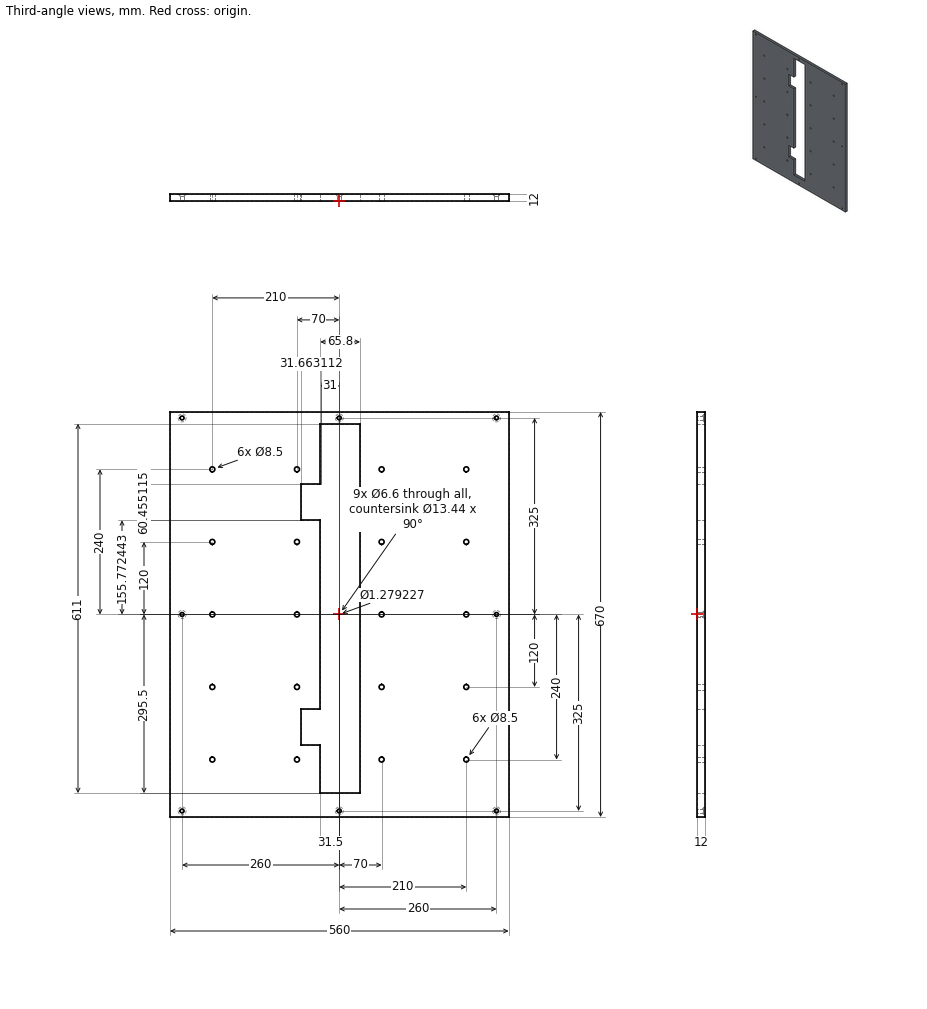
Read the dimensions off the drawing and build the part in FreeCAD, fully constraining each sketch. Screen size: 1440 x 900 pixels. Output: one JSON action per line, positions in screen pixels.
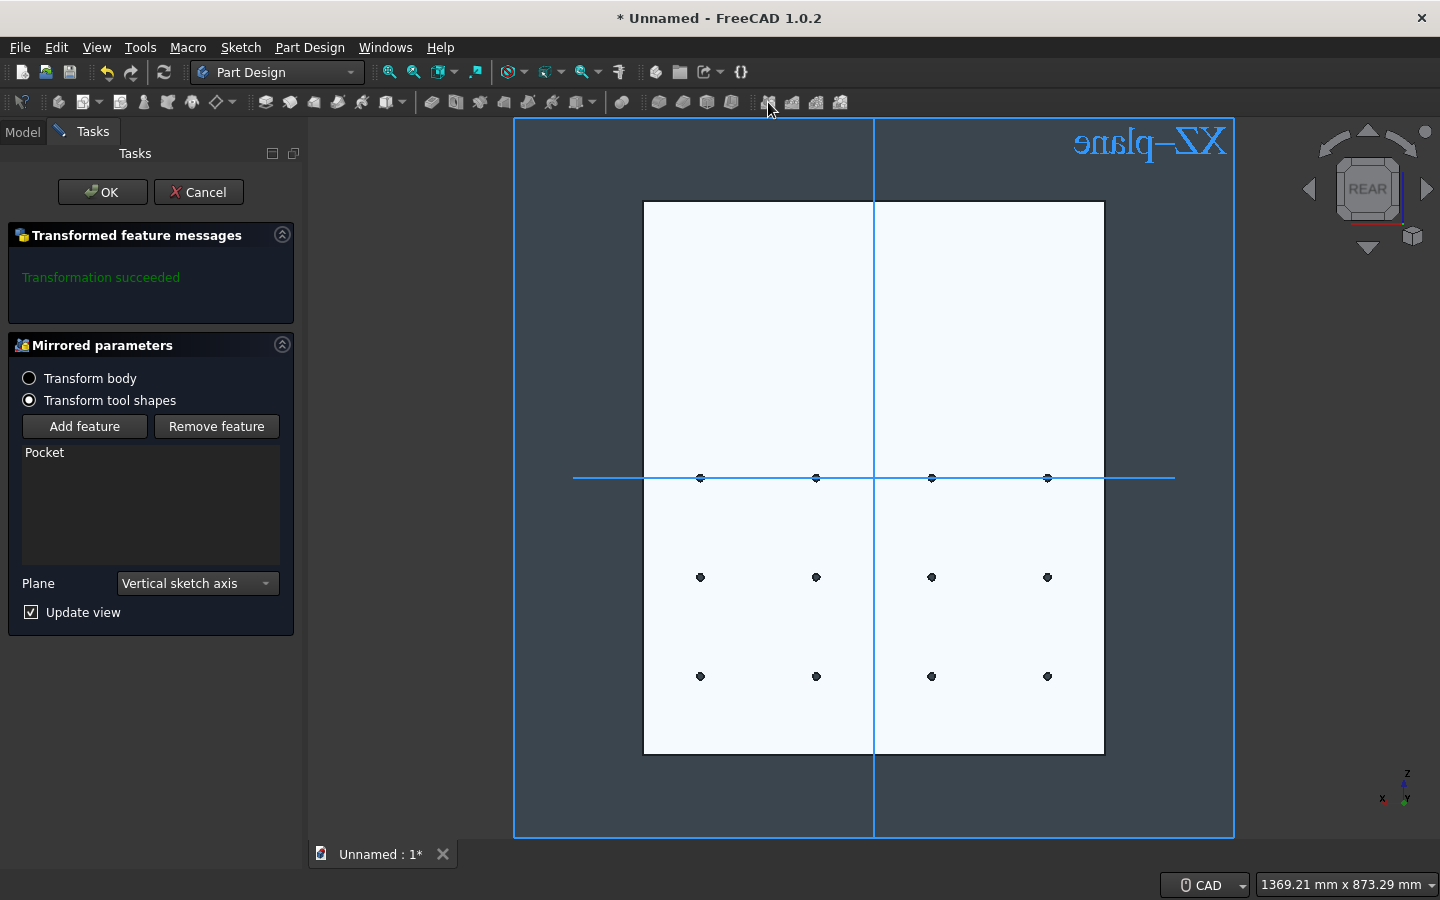
{"action": "left_click", "coordinate": [198, 584]}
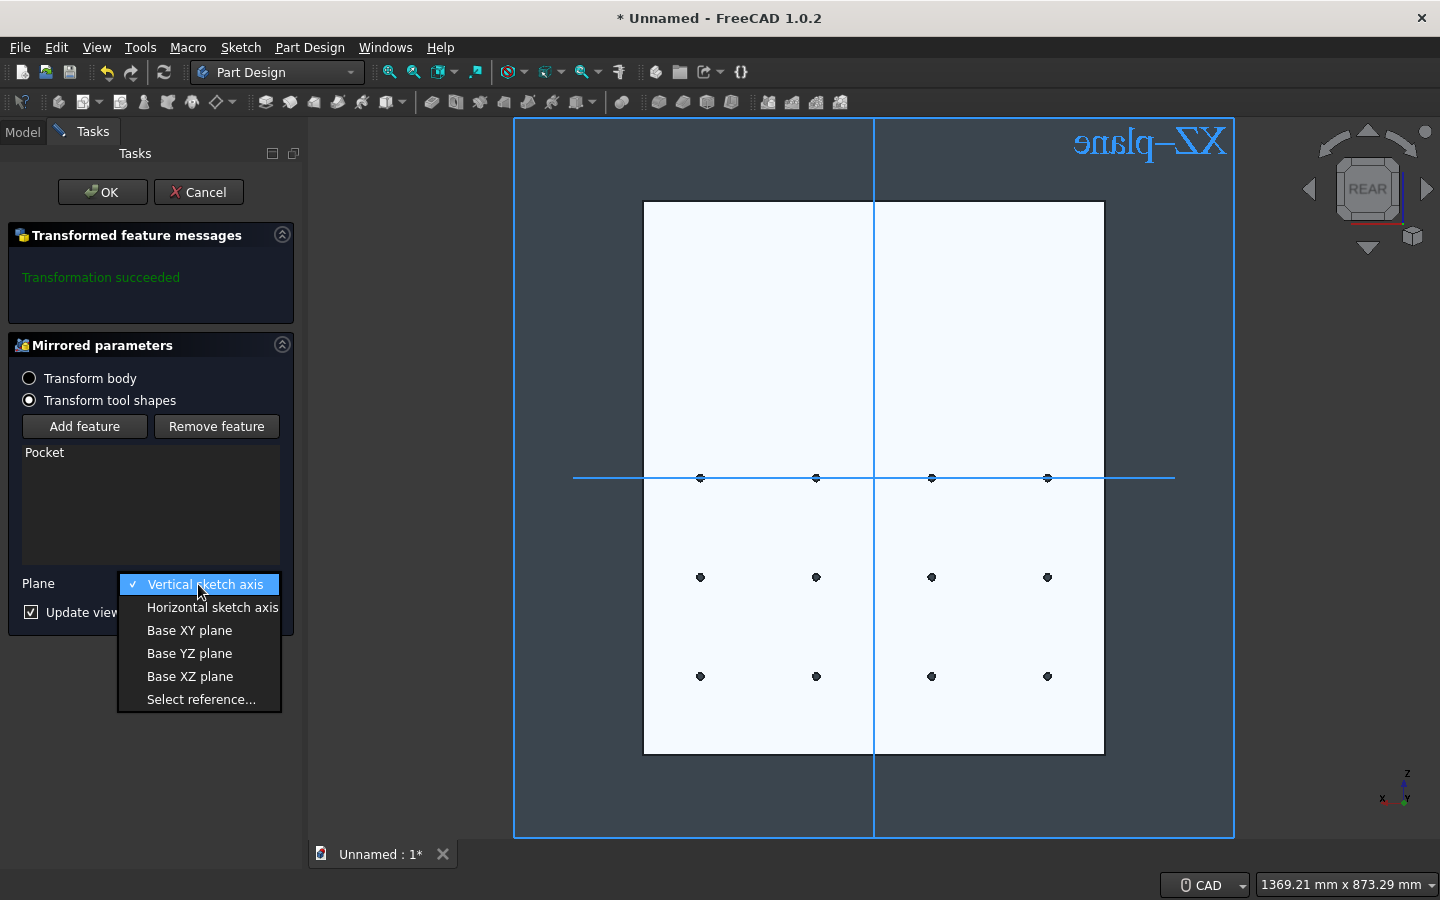
{"action": "left_click", "coordinate": [198, 630]}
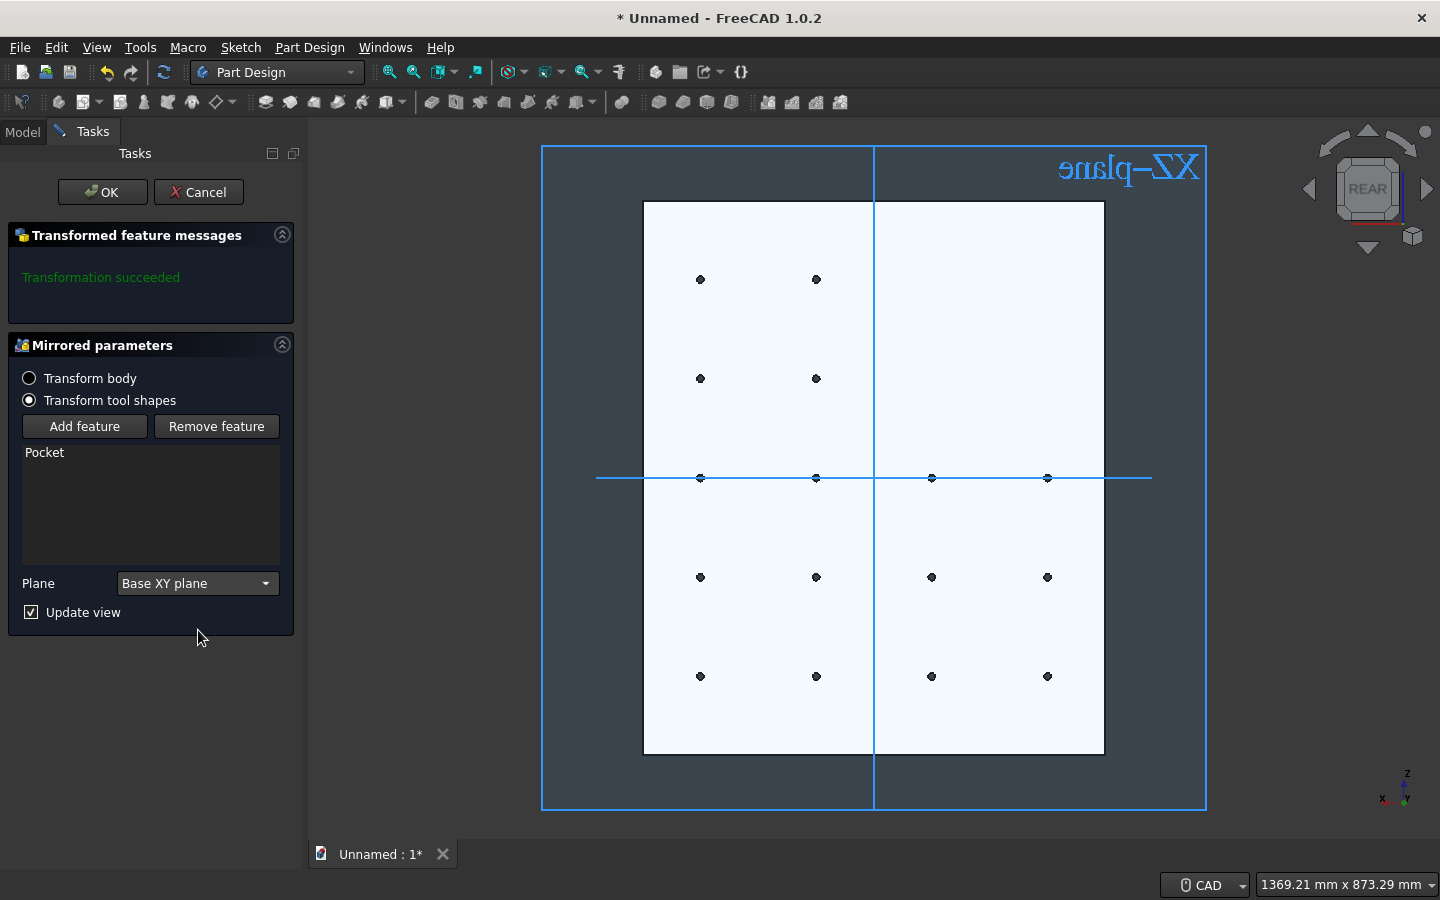
{"action": "left_click", "coordinate": [103, 192]}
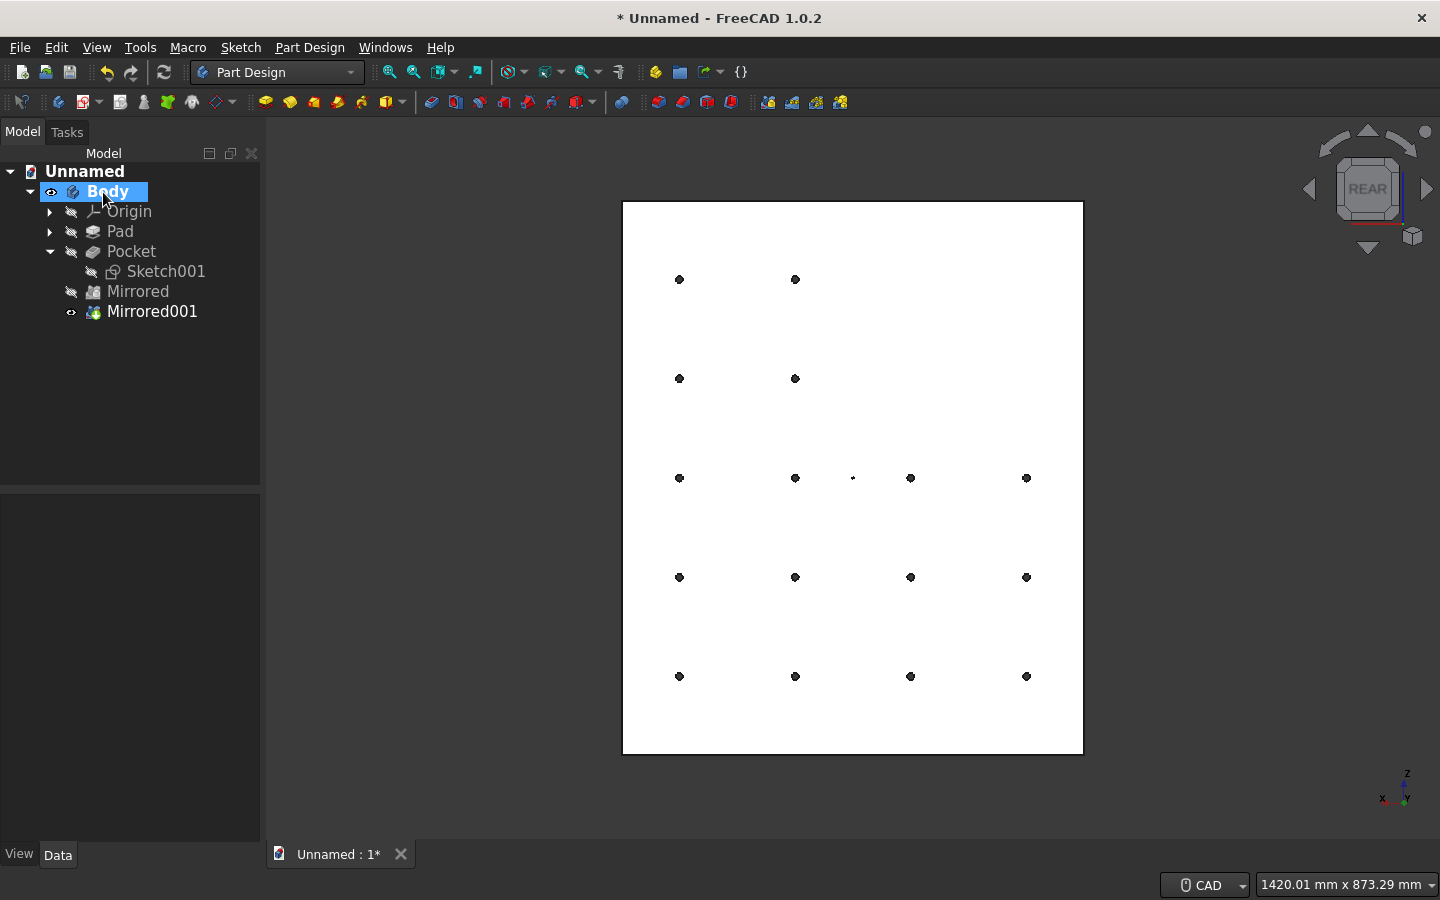
{"action": "left_click", "coordinate": [919, 319]}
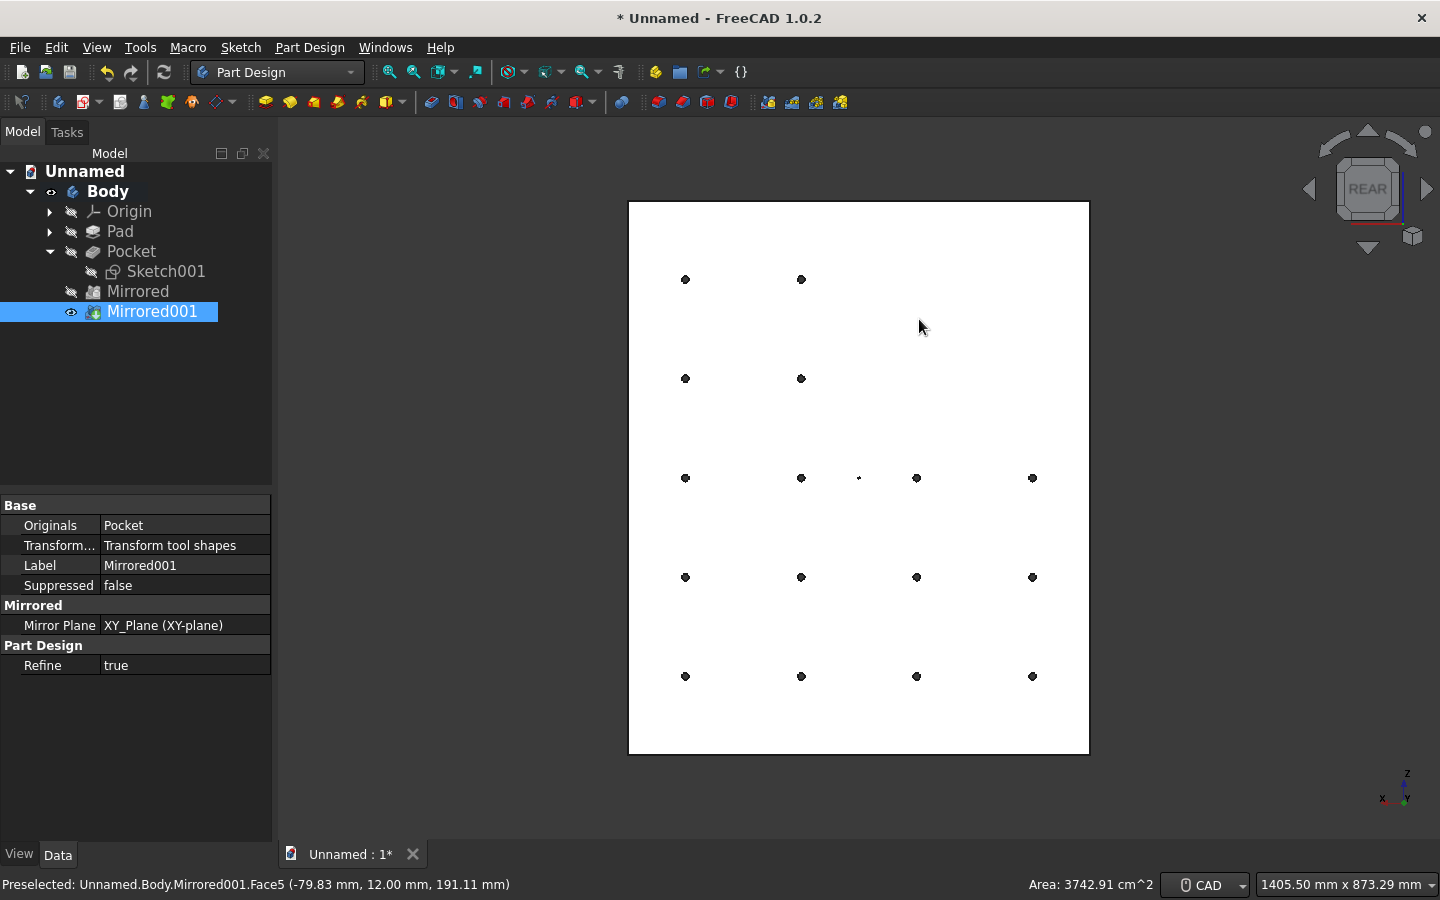
{"action": "left_click", "coordinate": [84, 102]}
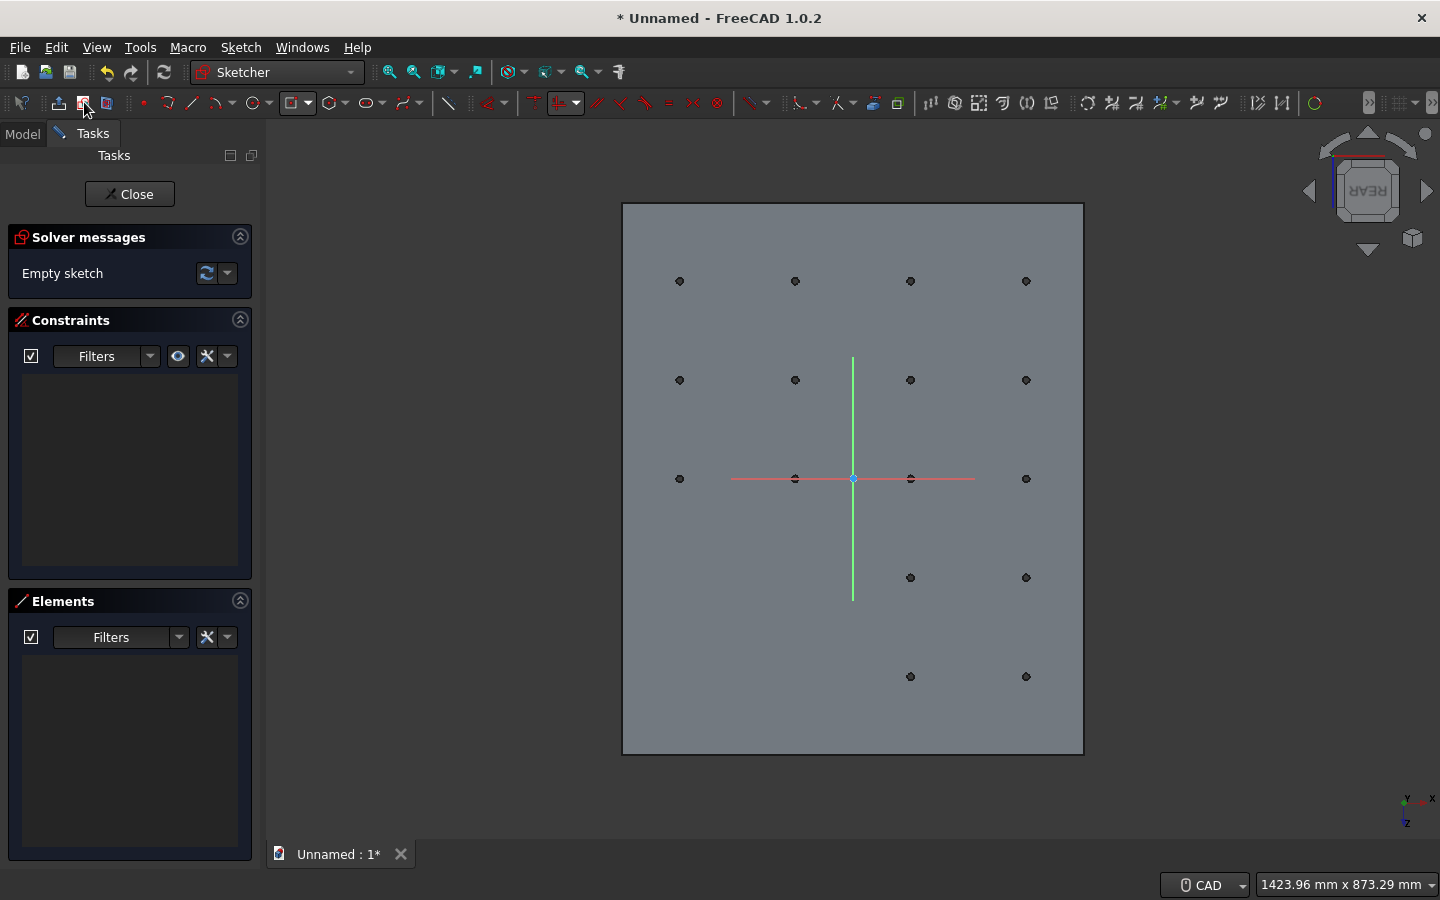
{"action": "scroll", "coordinate": [749, 659], "scroll_direction": "up", "scroll_amount": 4}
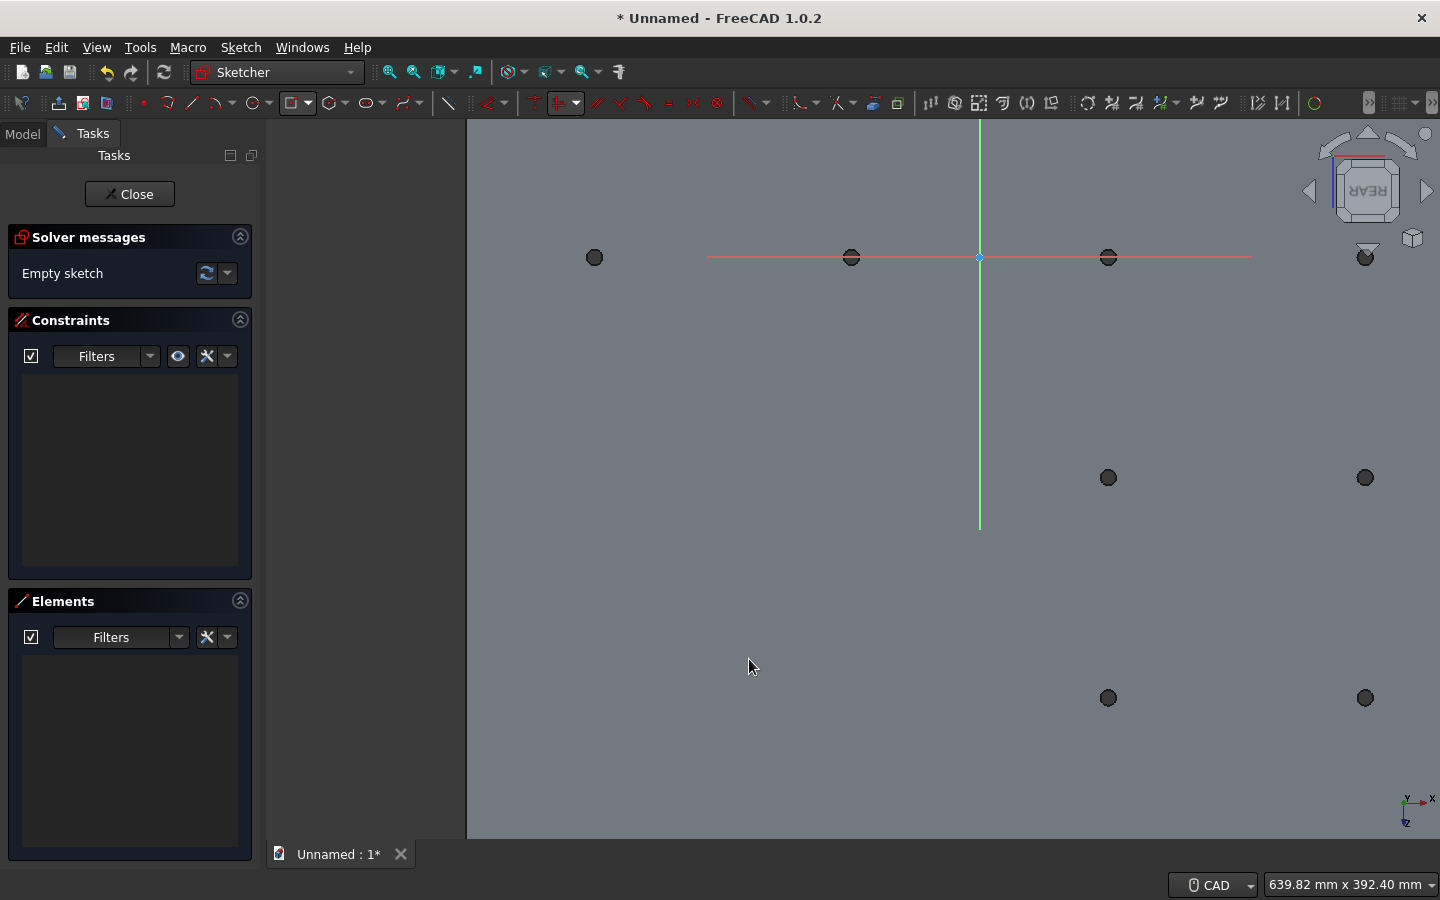
{"action": "left_click", "coordinate": [254, 104]}